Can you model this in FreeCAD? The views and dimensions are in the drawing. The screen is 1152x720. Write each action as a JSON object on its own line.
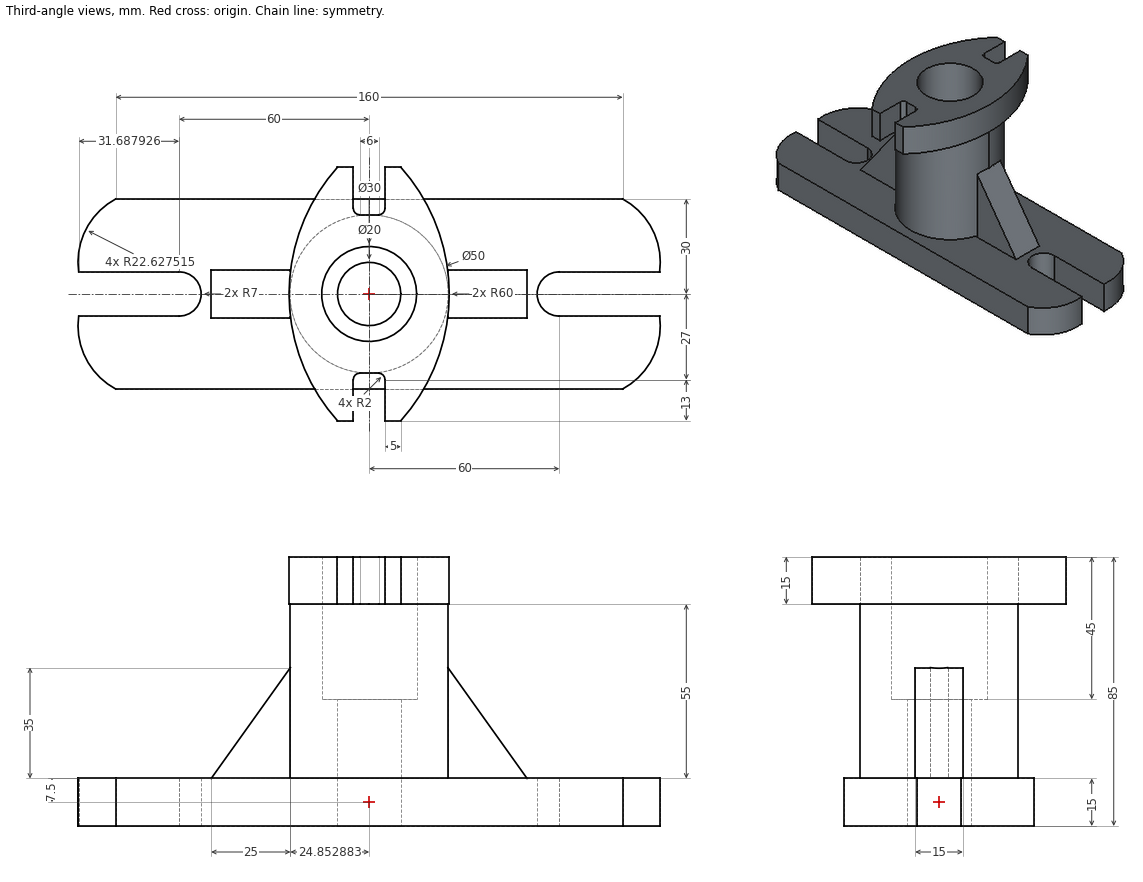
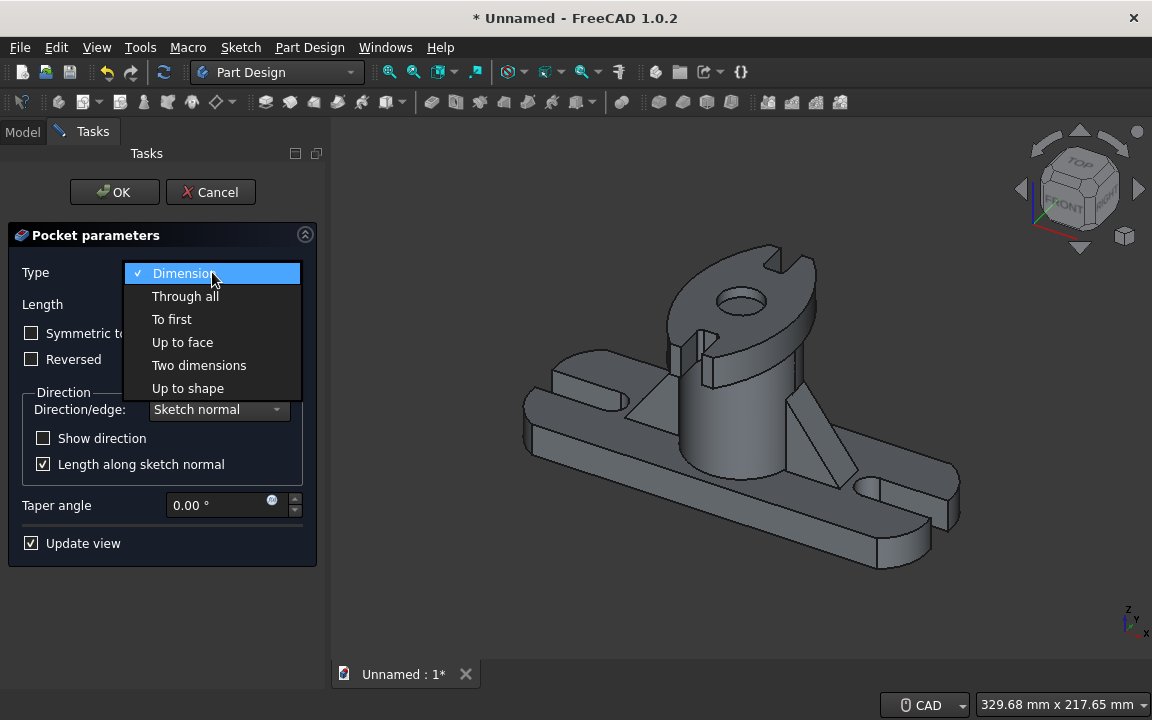
{"action": "left_click", "coordinate": [212, 296]}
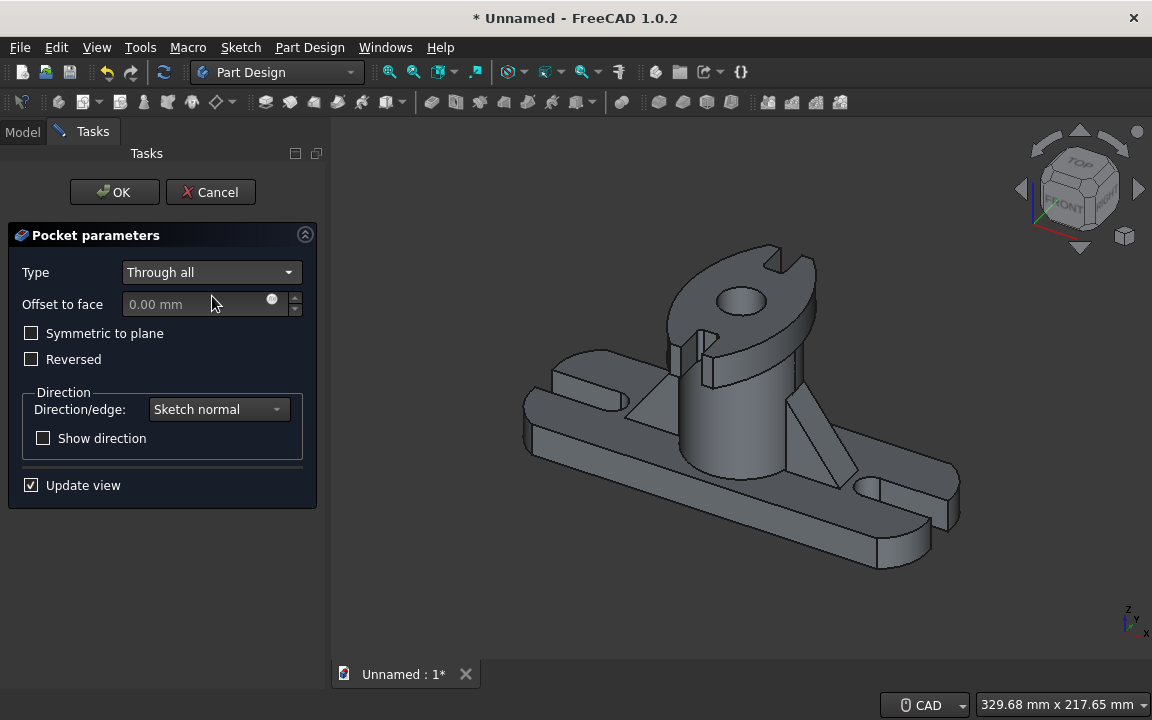
{"action": "left_click", "coordinate": [115, 192]}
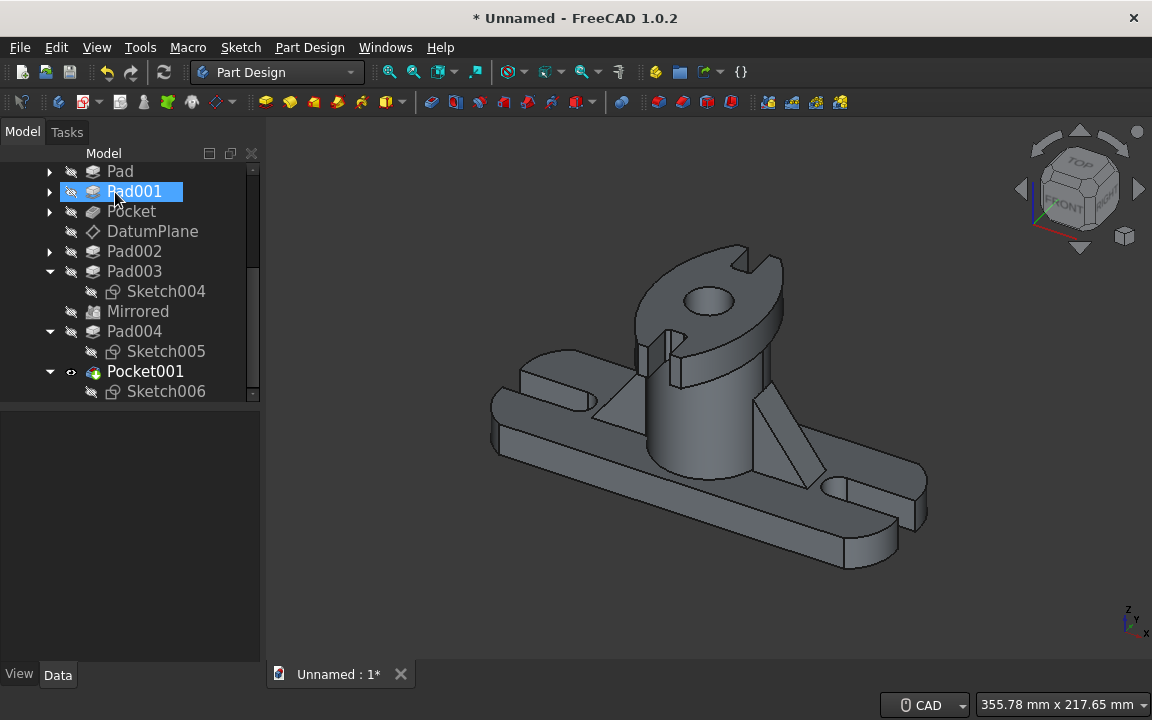
{"action": "left_click", "coordinate": [726, 325]}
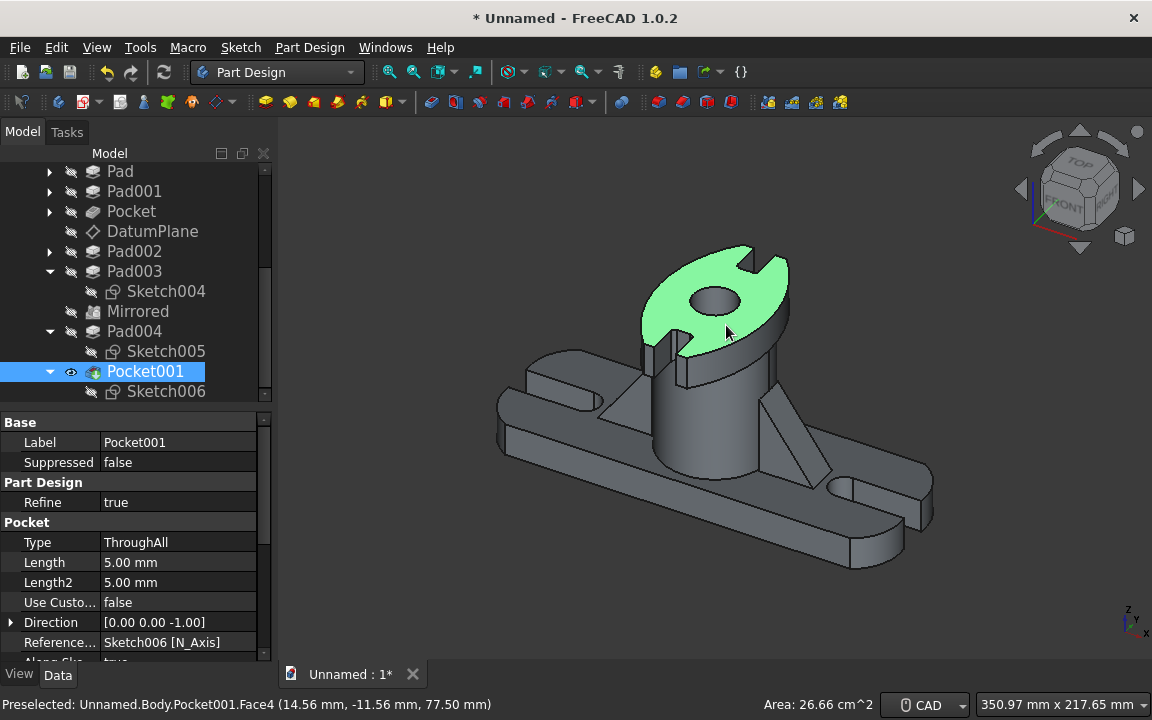
{"action": "left_click", "coordinate": [84, 102]}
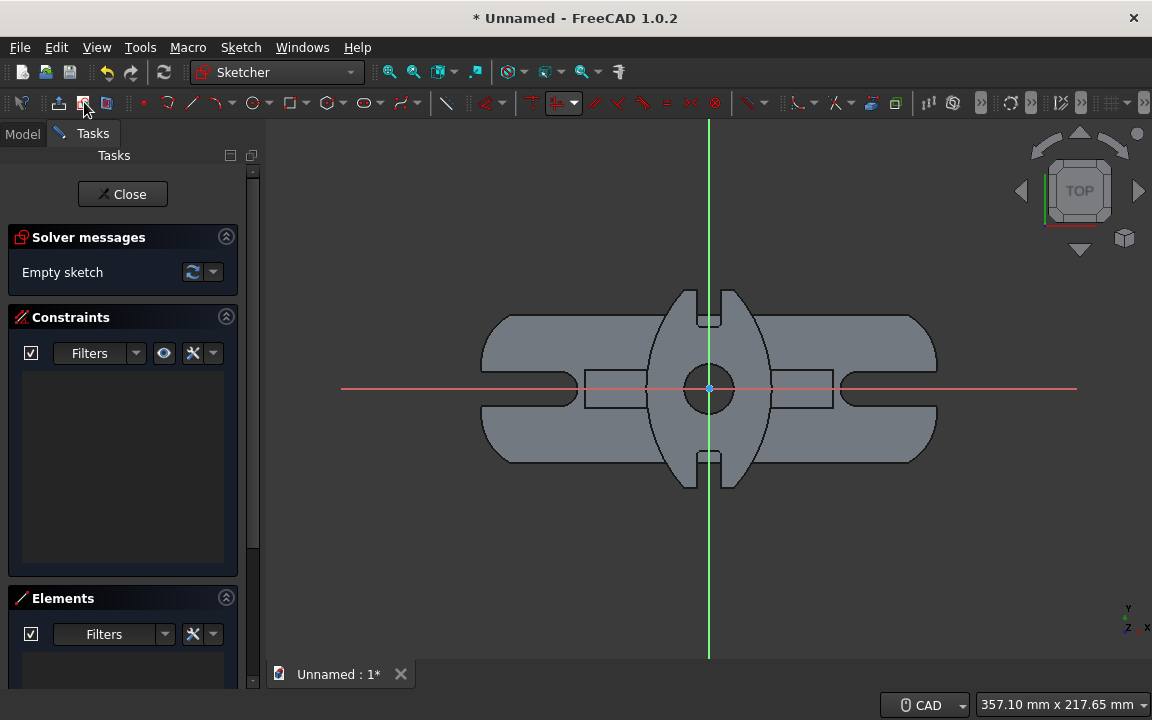
{"action": "scroll", "coordinate": [726, 389], "scroll_direction": "up", "scroll_amount": 8}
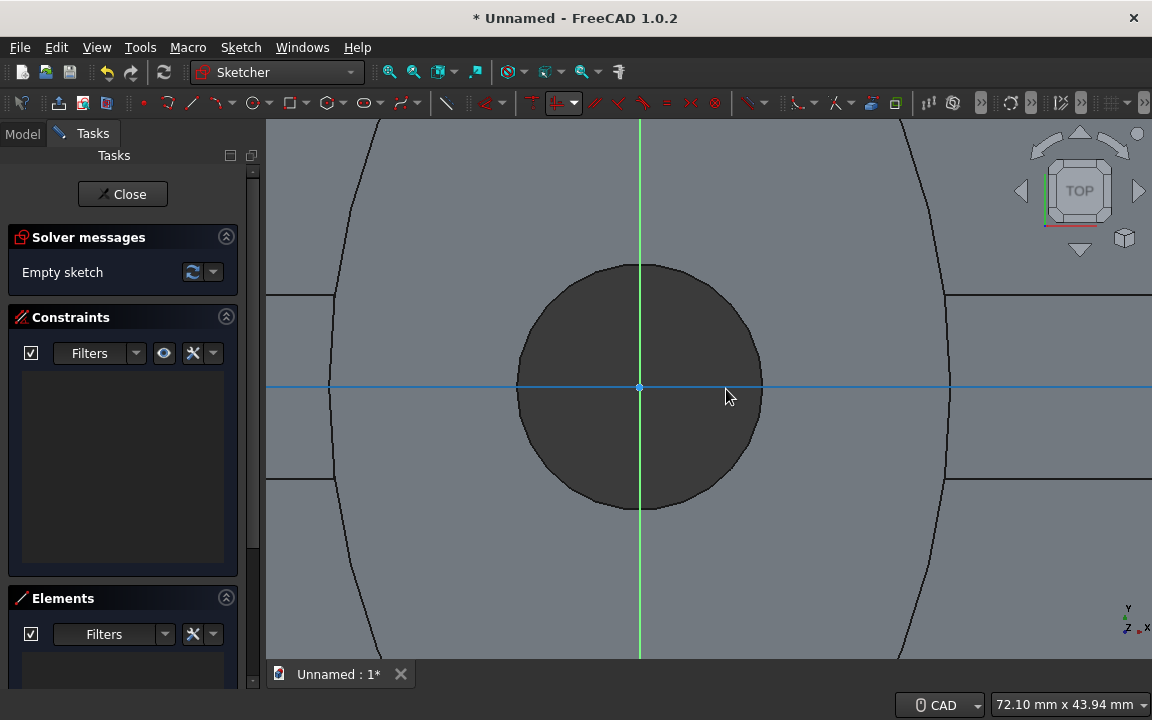
{"action": "key", "text": "g c"}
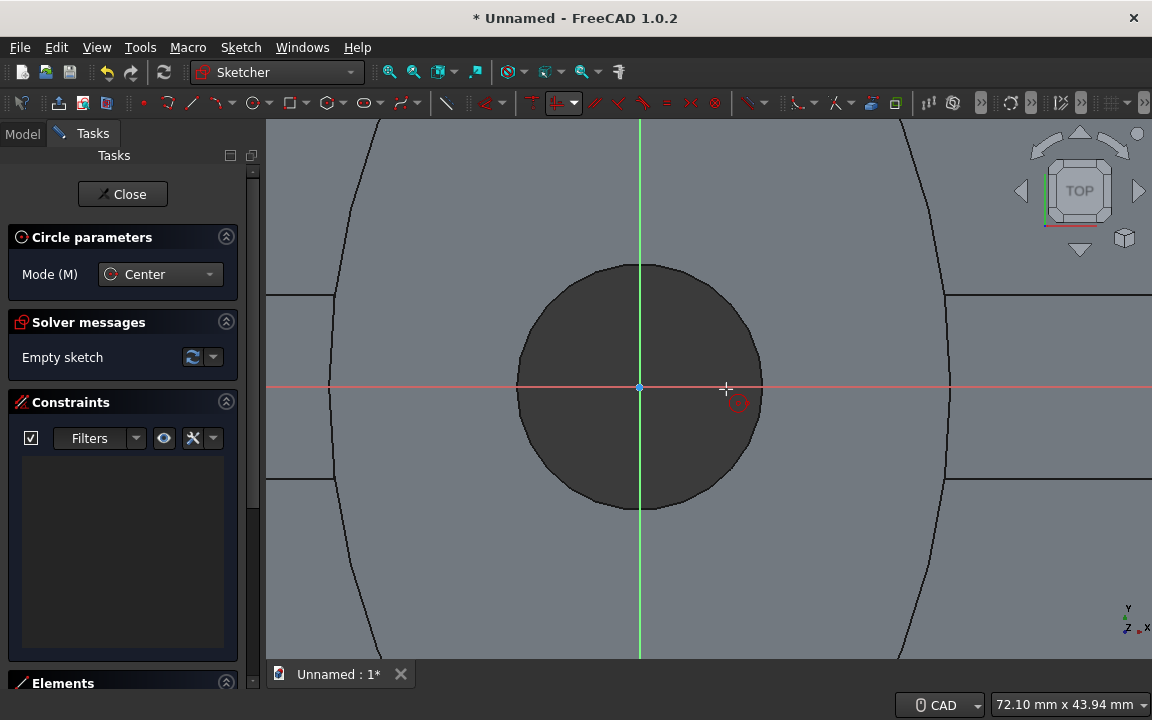
{"action": "left_click", "coordinate": [640, 387]}
{"action": "mouse_move", "coordinate": [770, 257]}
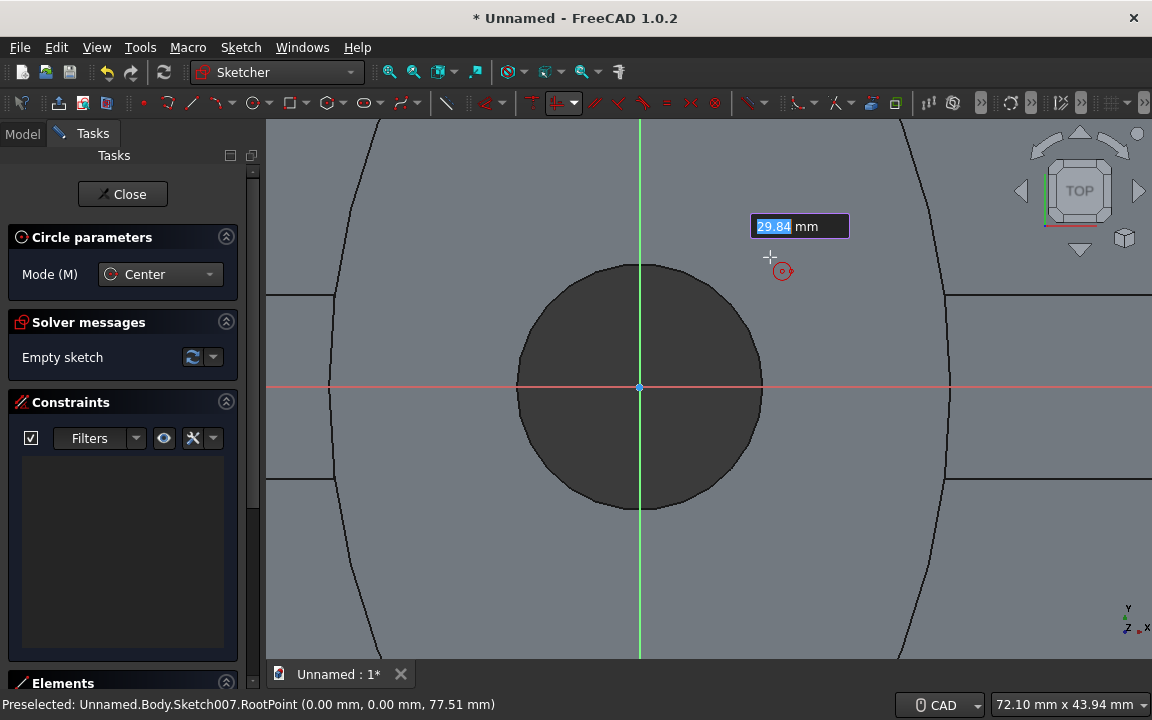
{"action": "type", "text": "30"}
{"action": "key", "text": "Return"}
{"action": "key", "text": "Escape"}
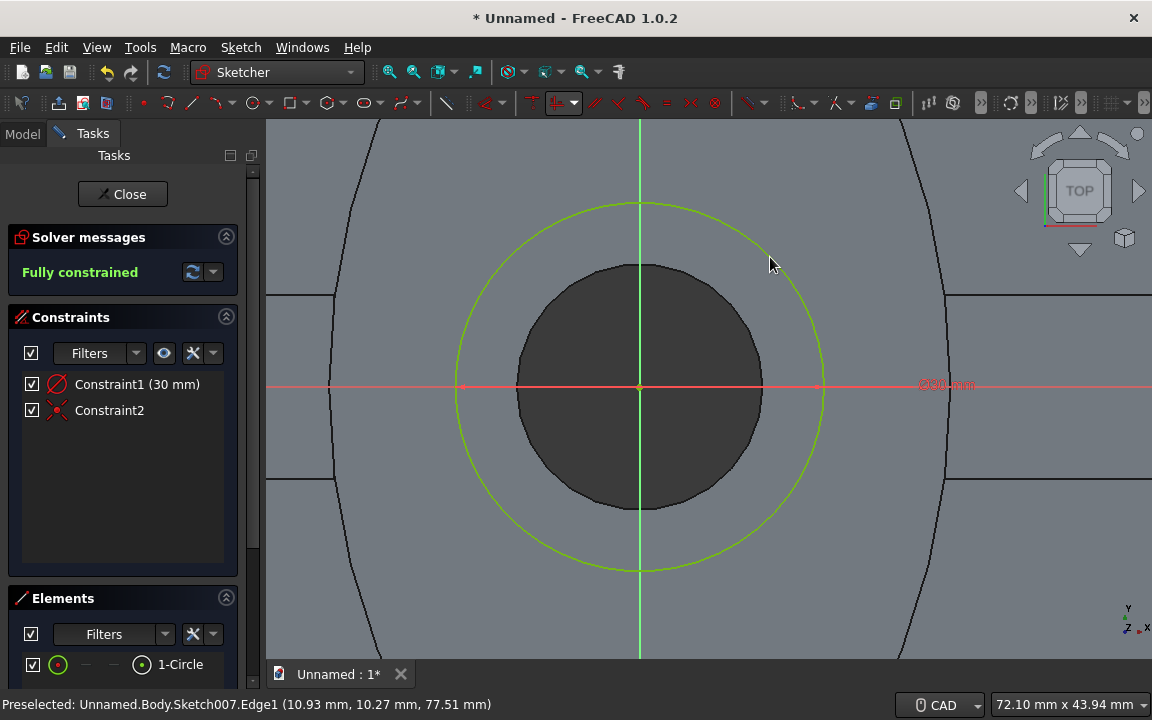
{"action": "left_click", "coordinate": [123, 194]}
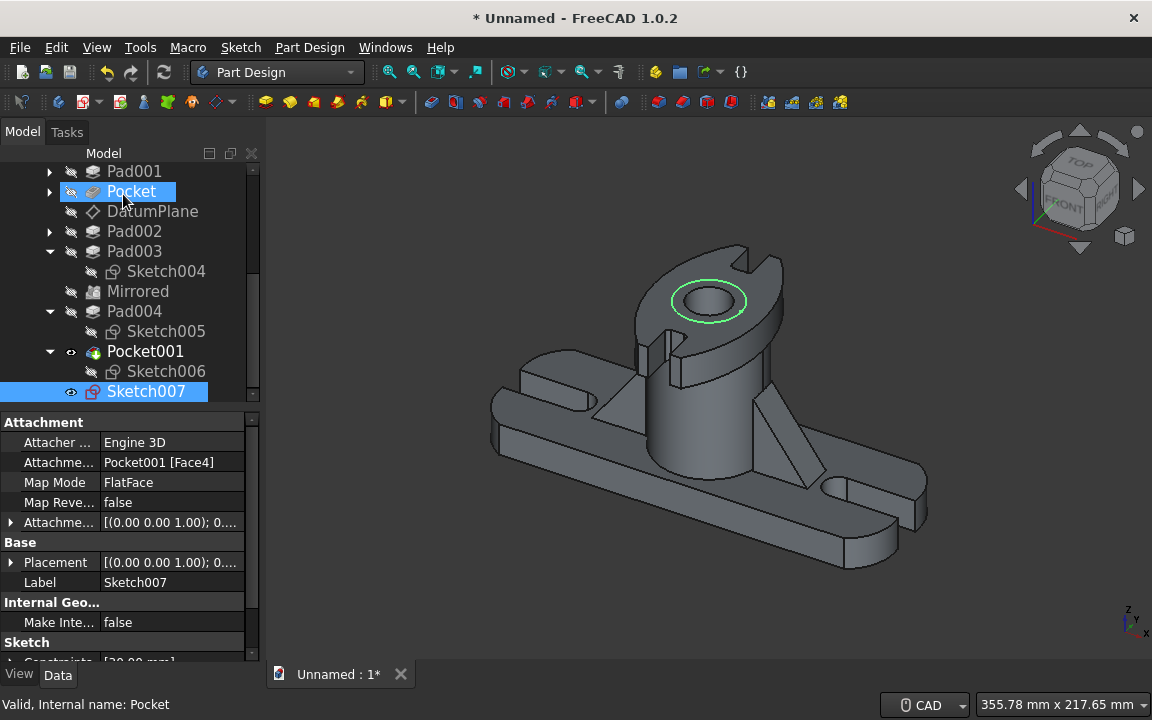
{"action": "left_click", "coordinate": [432, 102]}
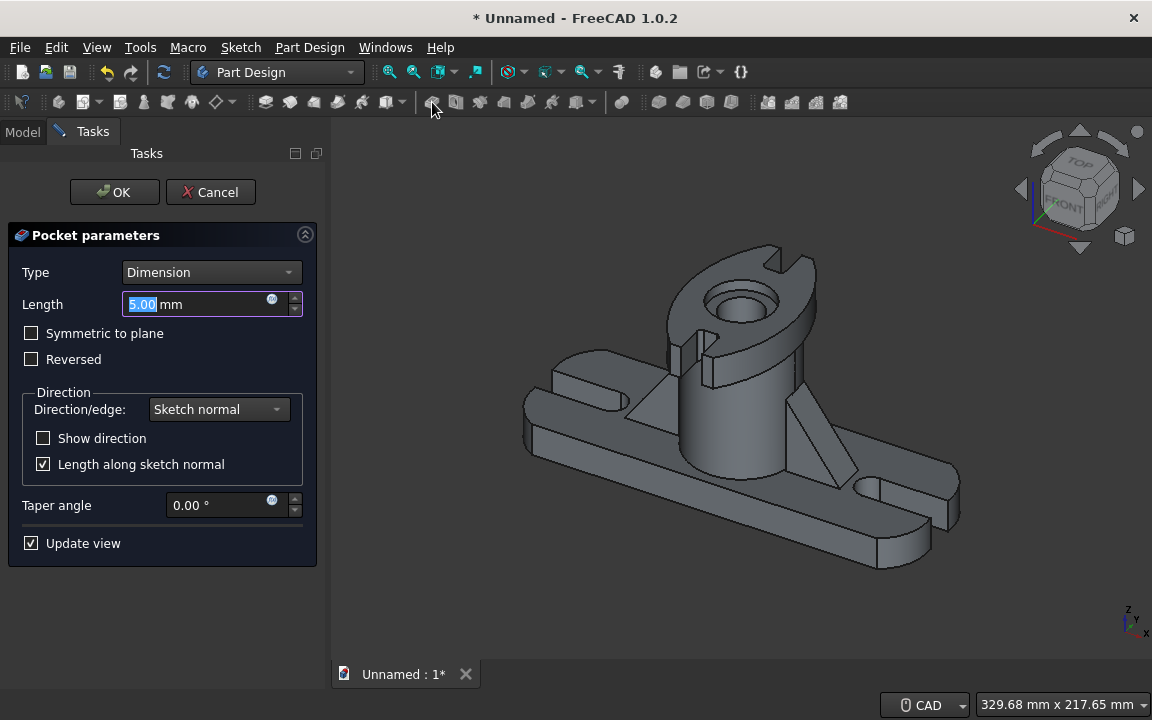
{"action": "type", "text": "45"}
{"action": "key", "text": "Tab"}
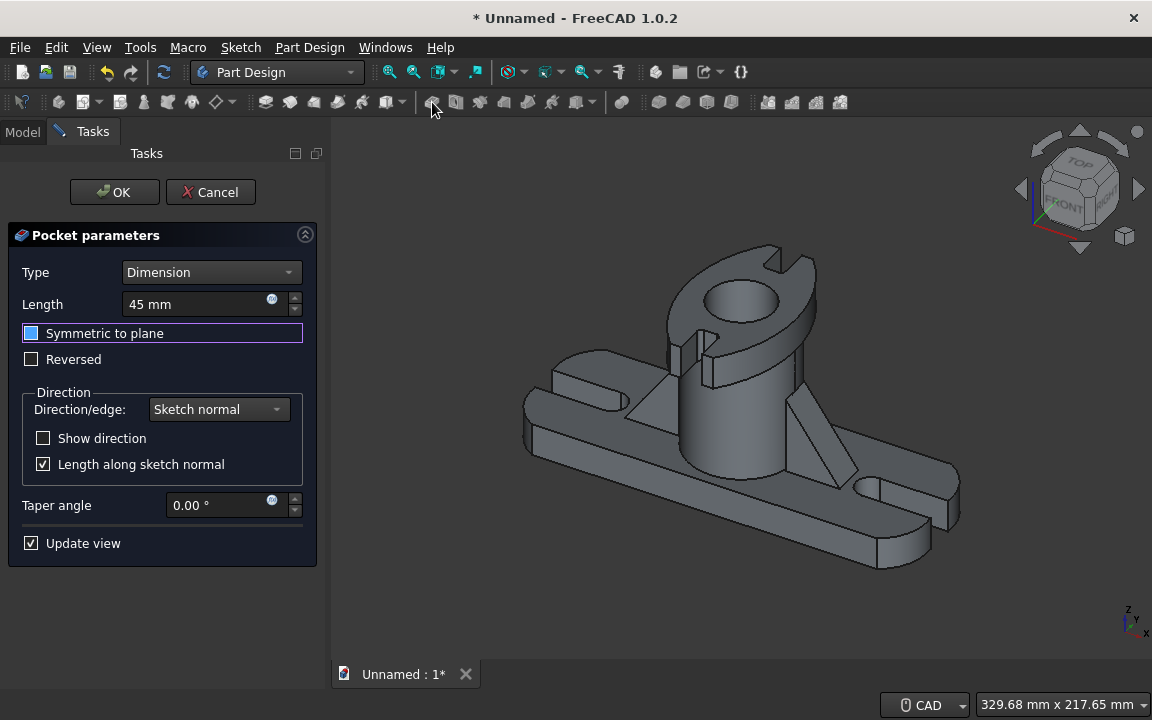
{"action": "left_click", "coordinate": [115, 192]}